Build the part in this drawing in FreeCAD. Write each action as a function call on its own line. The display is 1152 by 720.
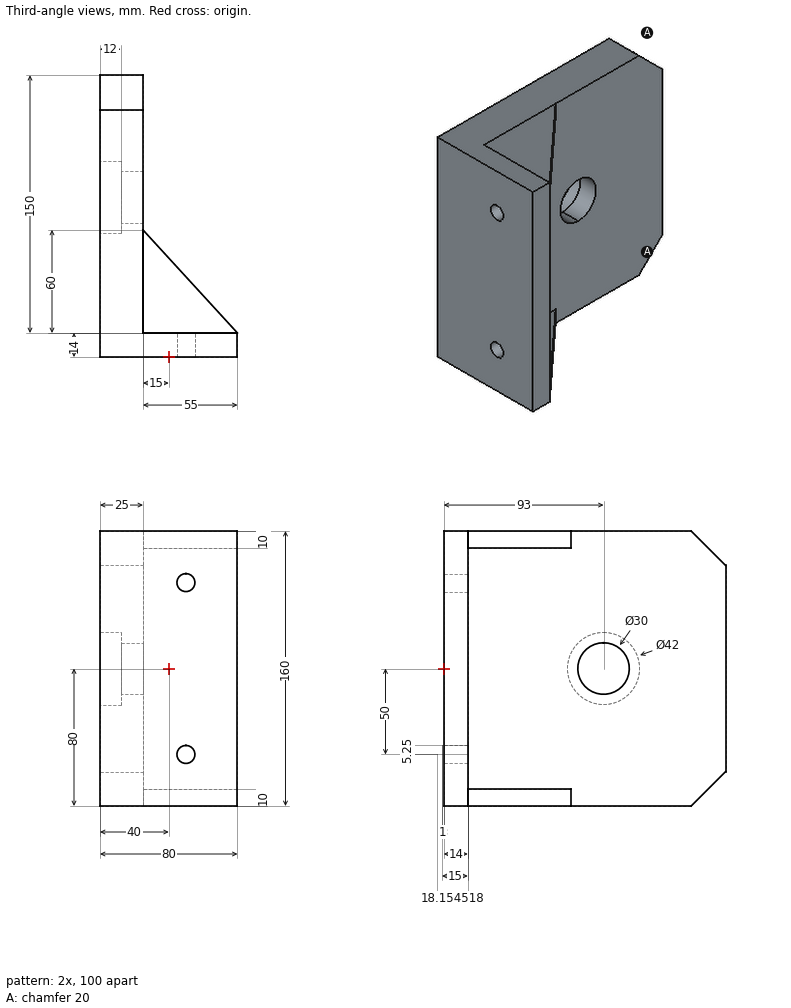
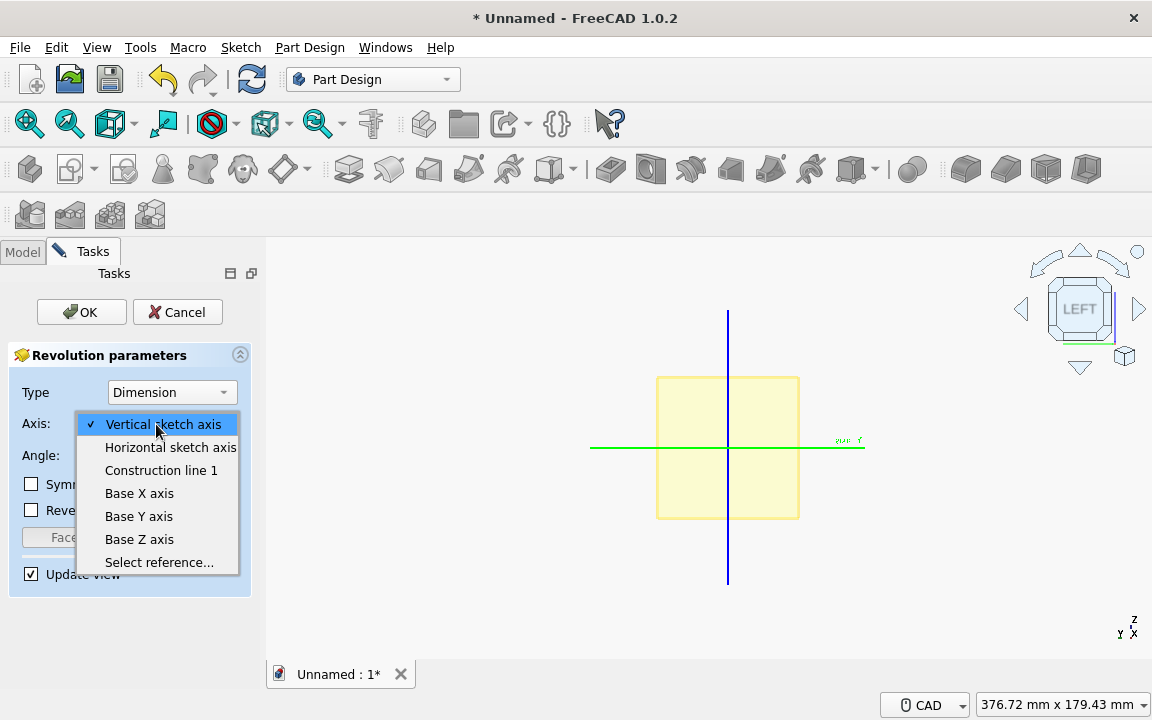
click(156, 470)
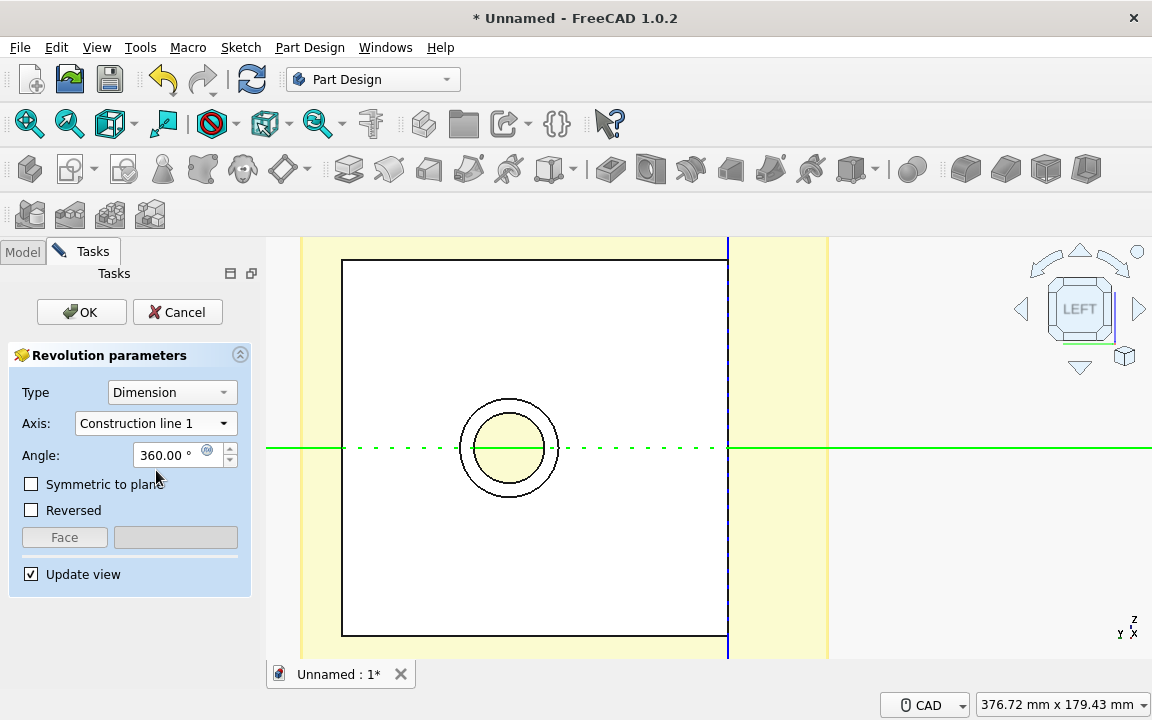
click(82, 312)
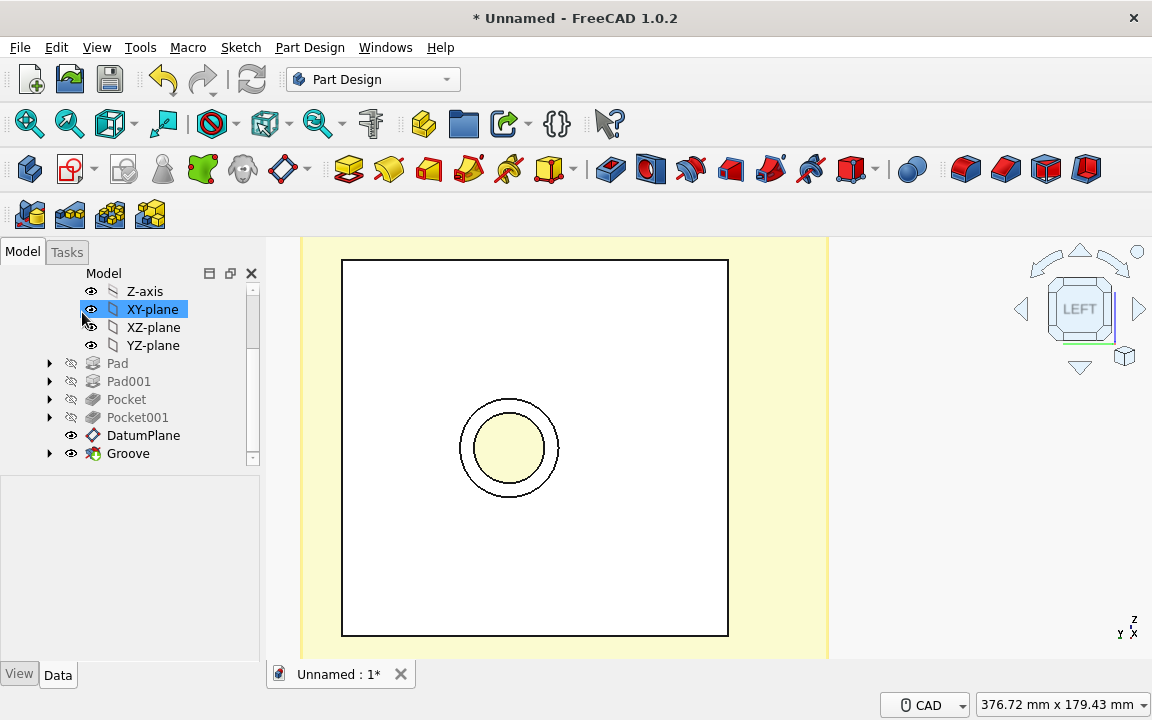
click(116, 435)
key(space)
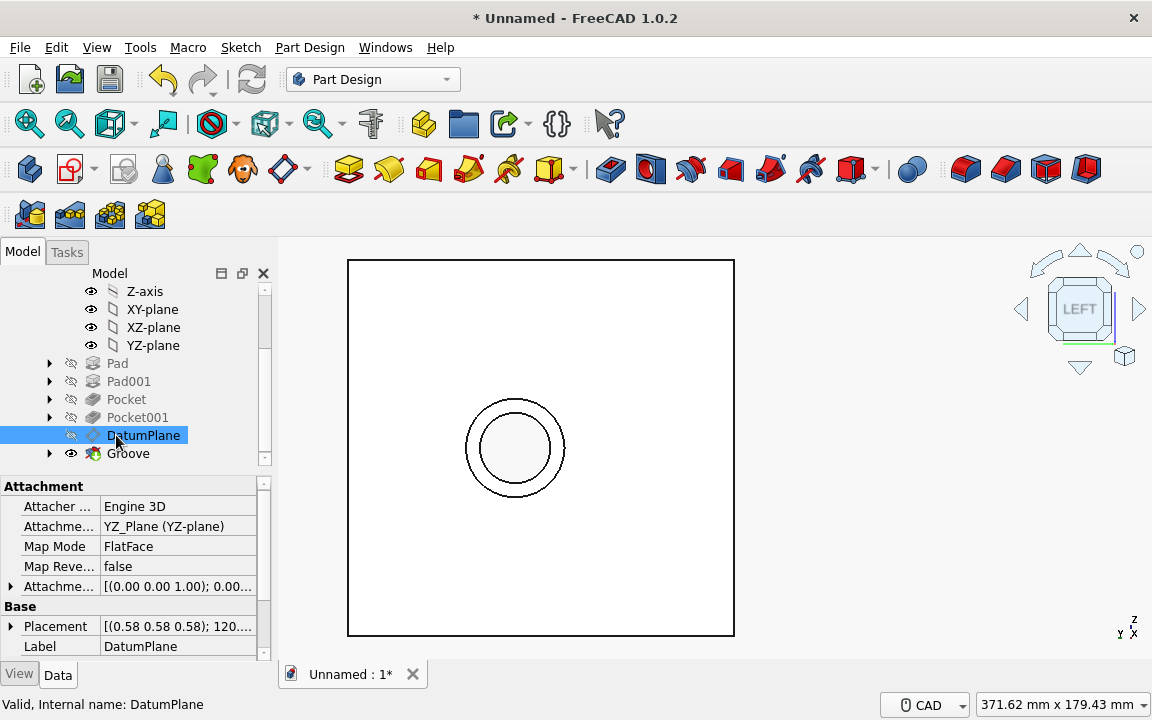
click(116, 453)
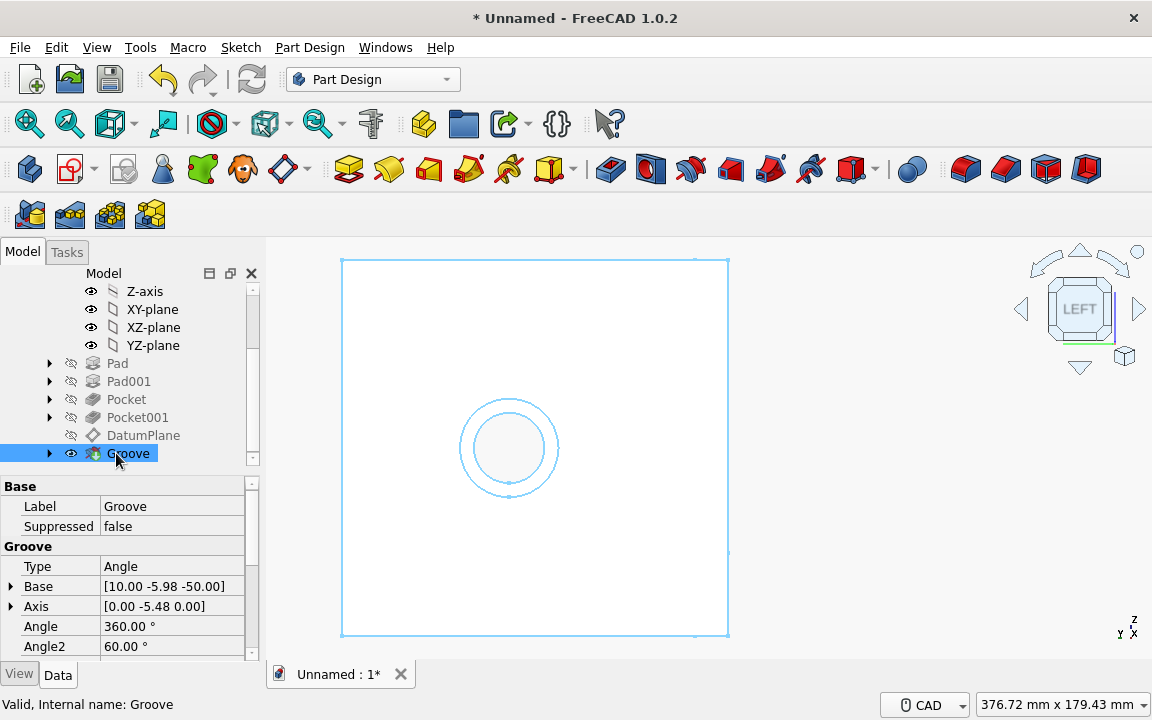
click(70, 214)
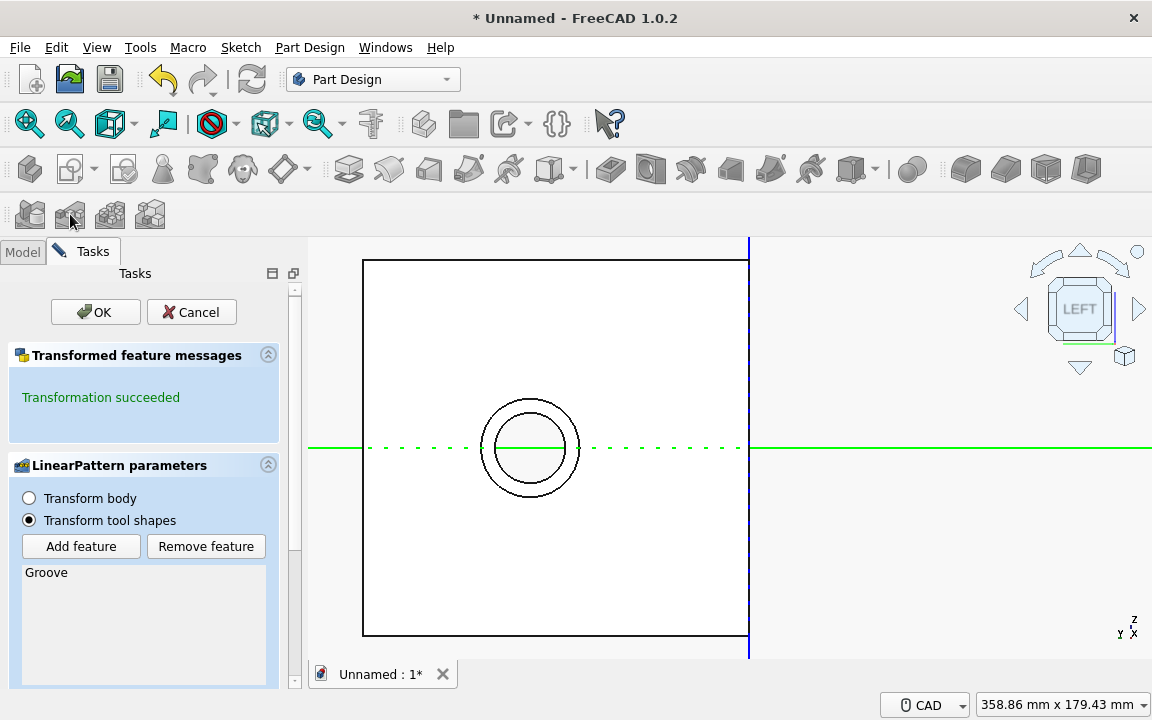
scroll(295, 486, down, 2)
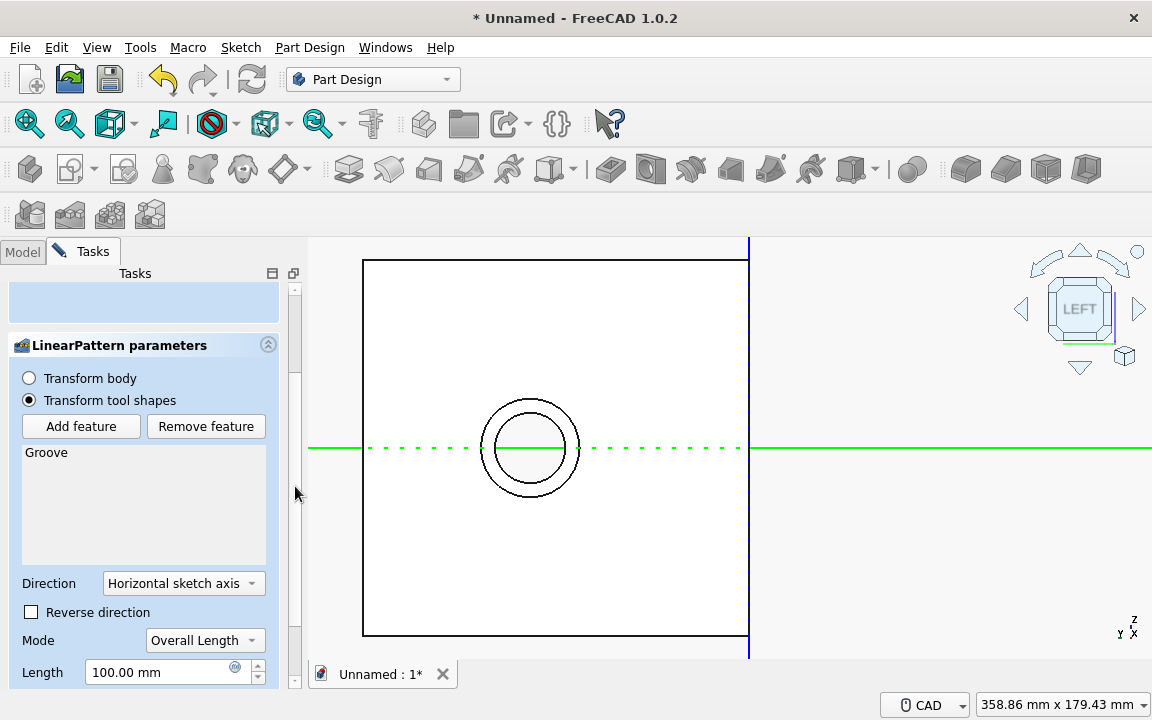
click(184, 584)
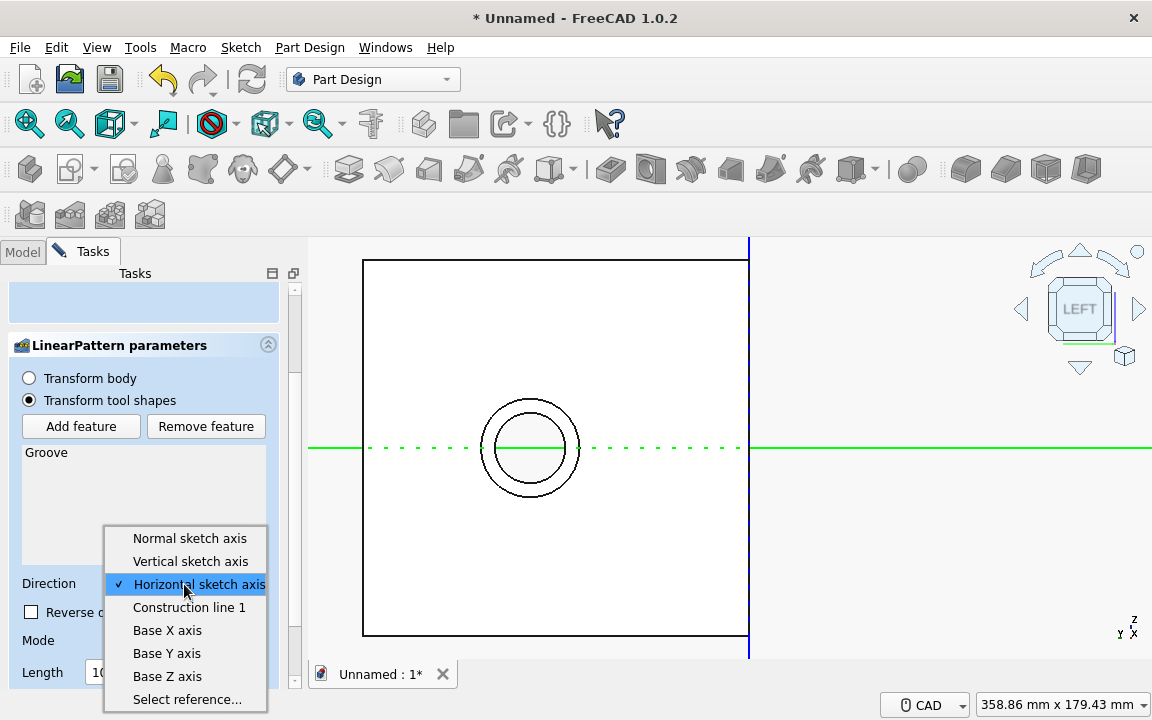
click(184, 676)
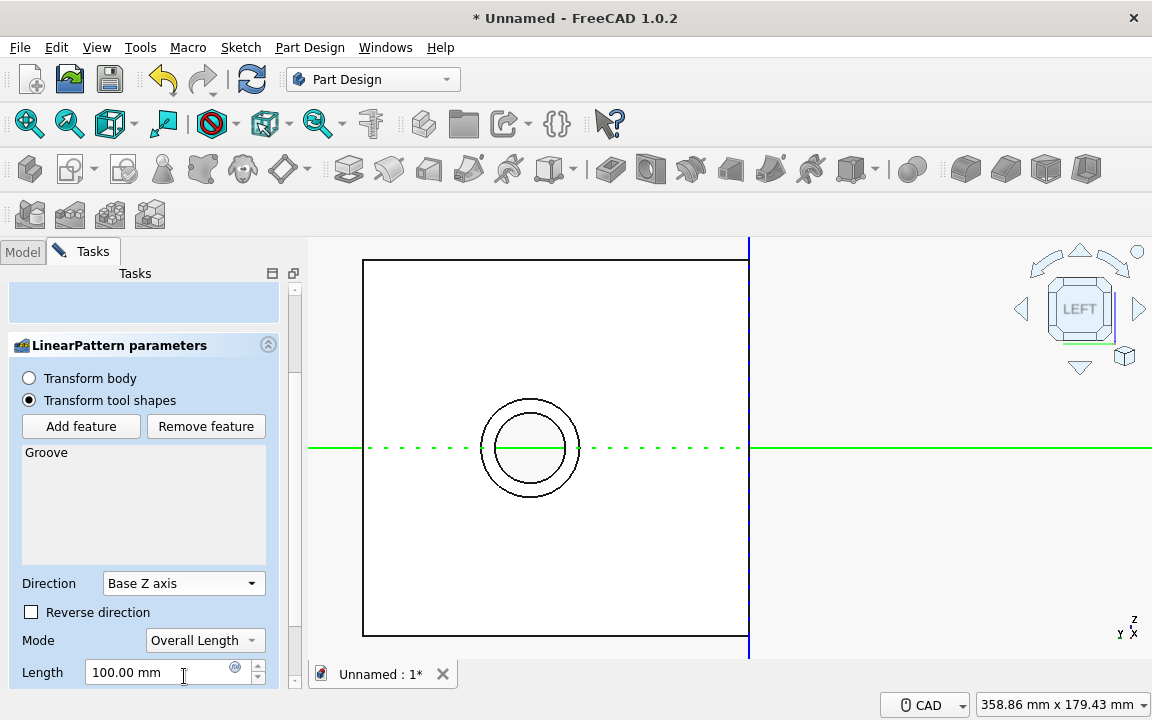
click(206, 640)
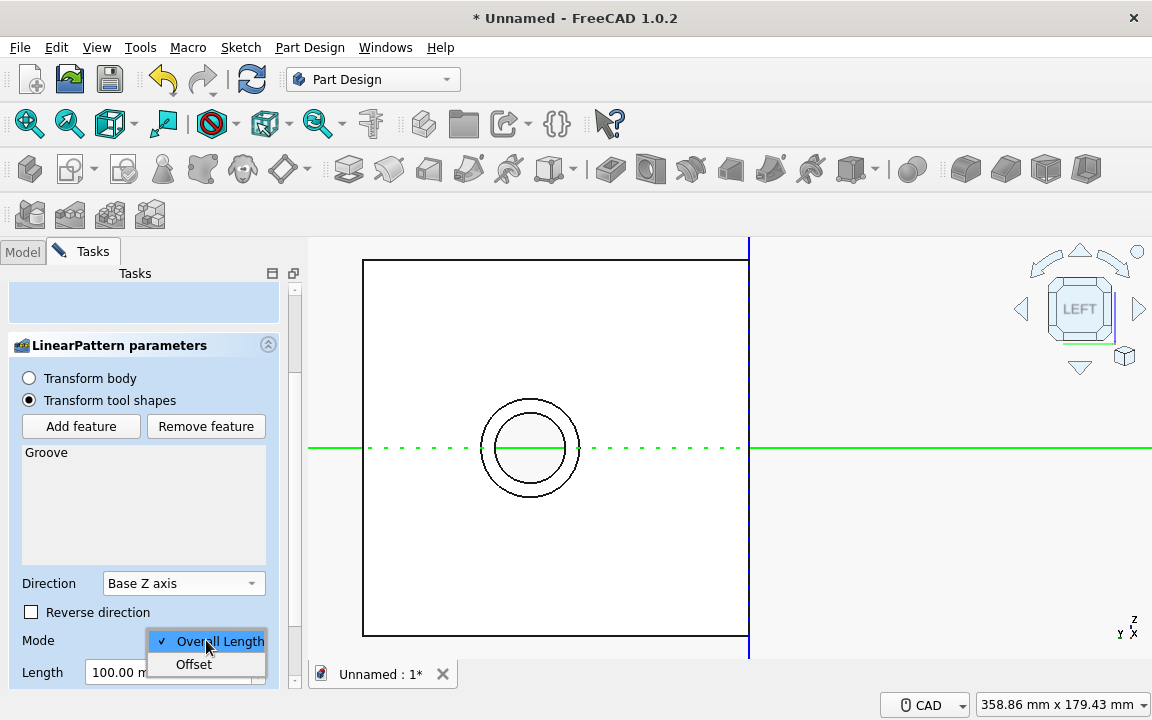
click(206, 664)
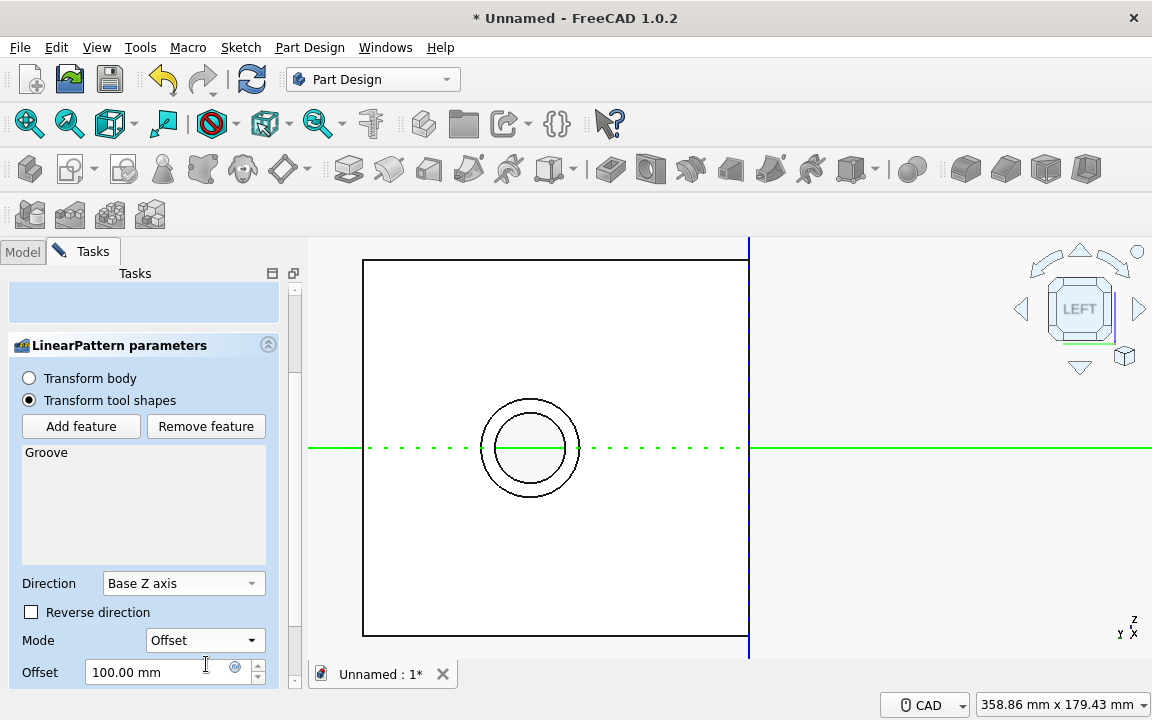
triple_click(168, 672)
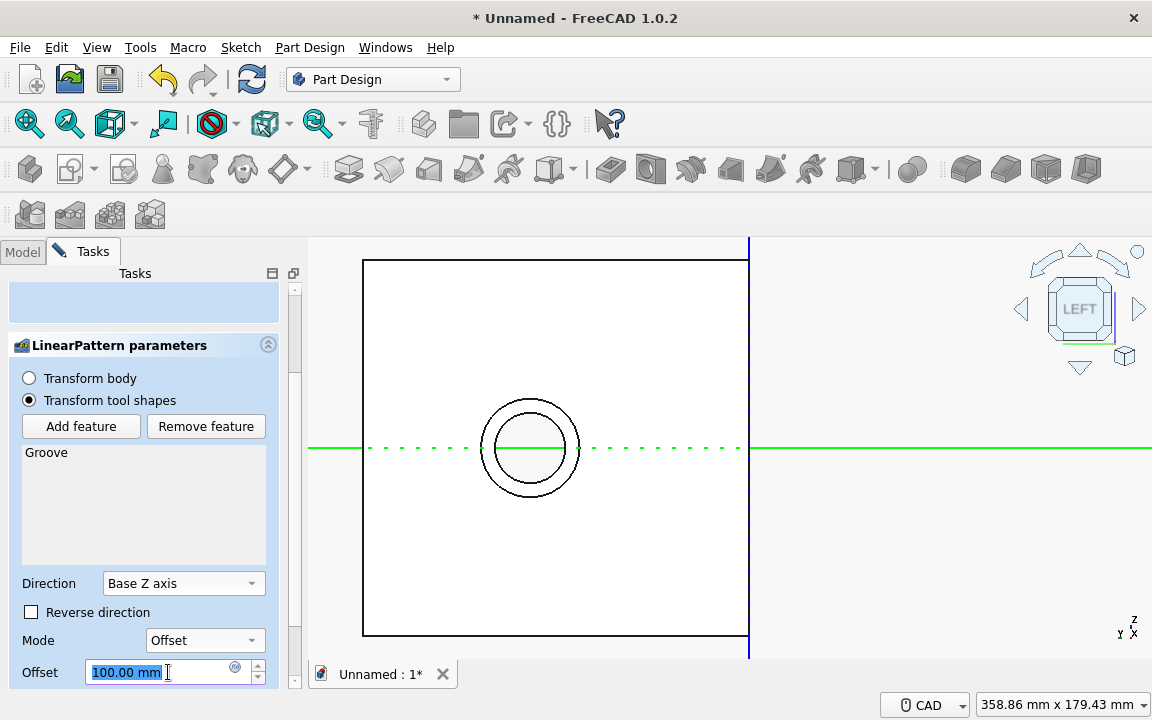
text(100)
key(Tab)